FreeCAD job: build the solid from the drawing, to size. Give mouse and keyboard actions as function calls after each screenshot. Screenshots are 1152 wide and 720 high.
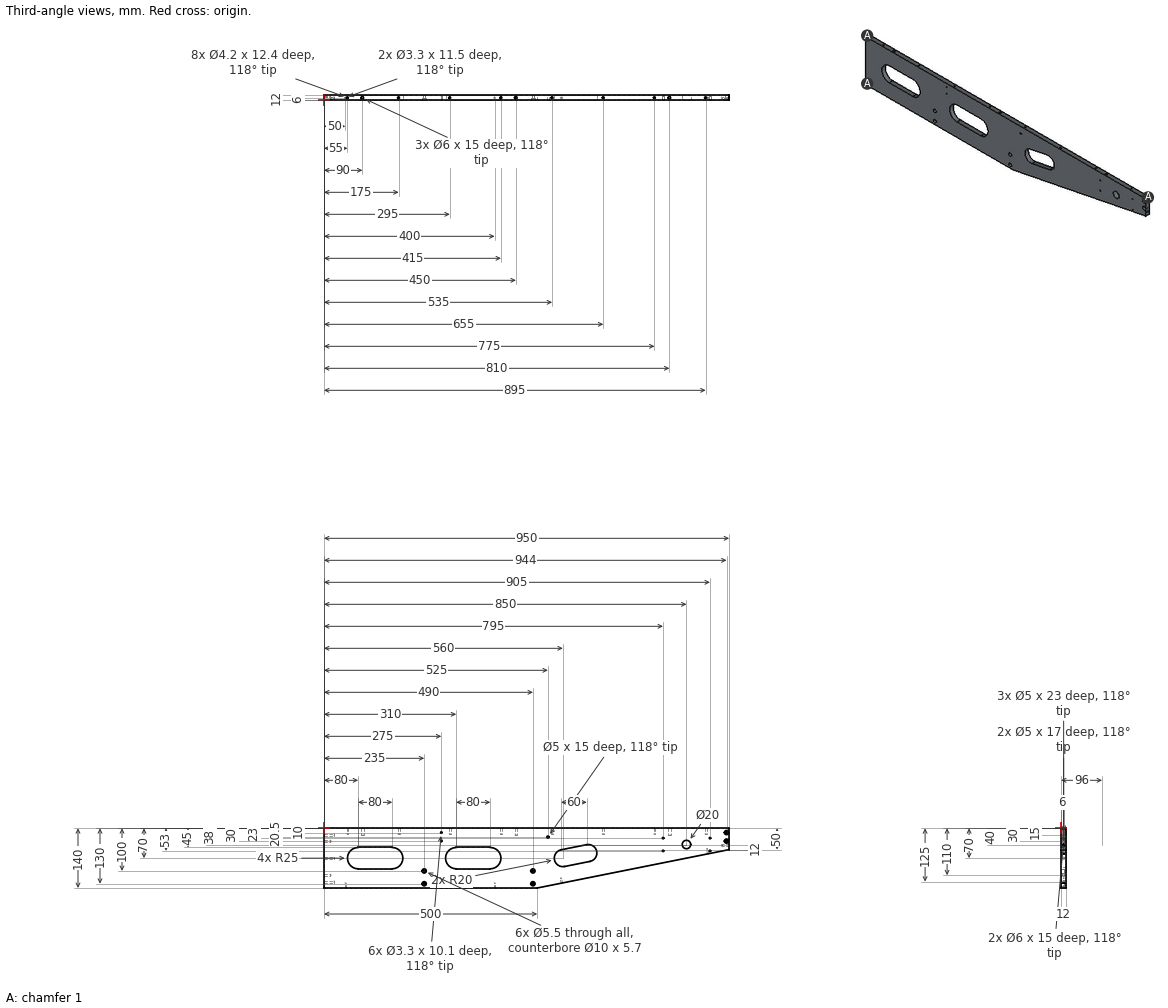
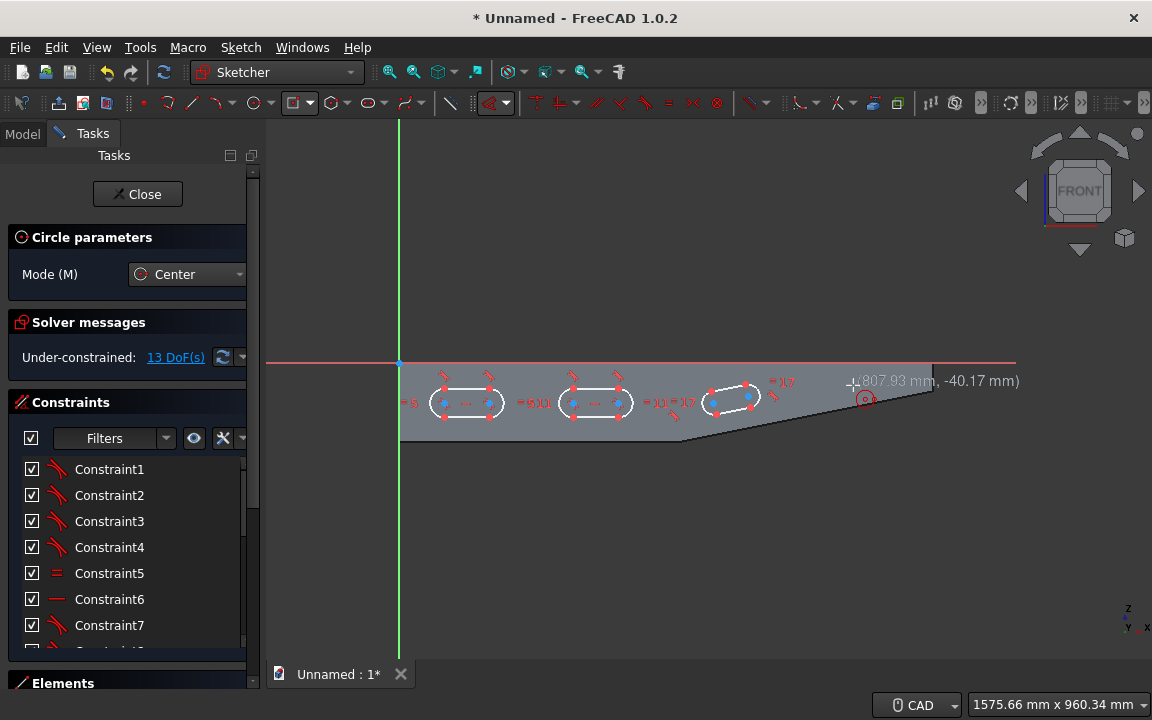
click(877, 384)
move(881, 380)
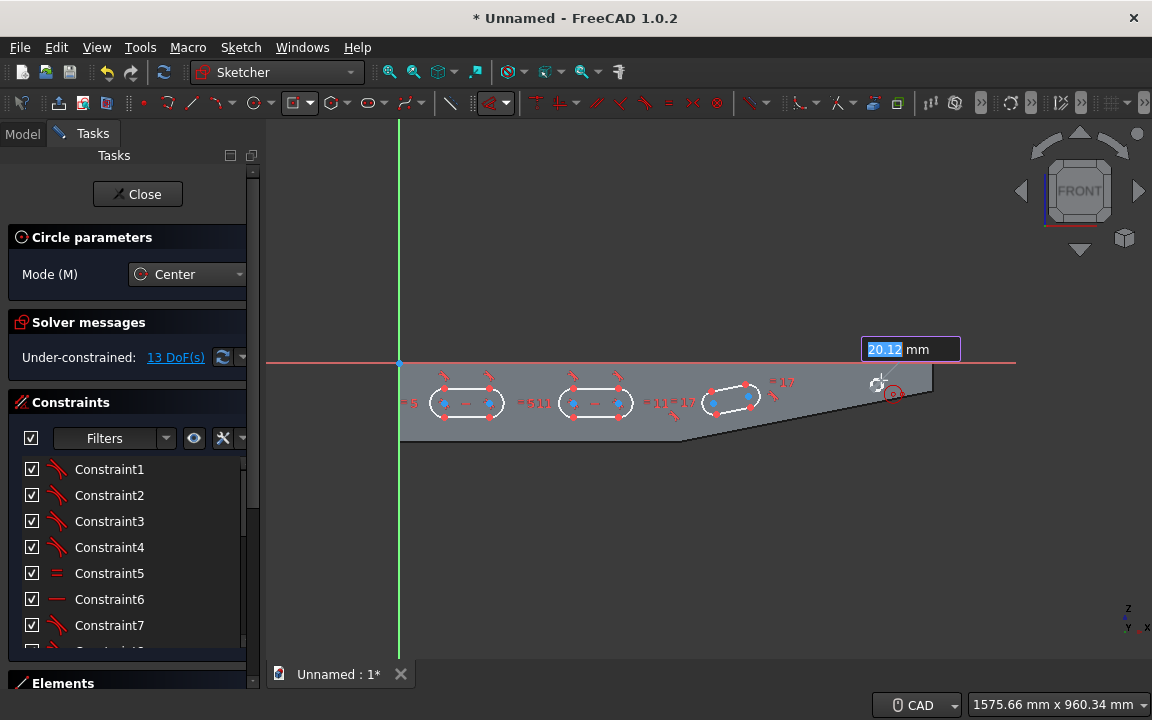
text(20)
key(Return)
key(Escape)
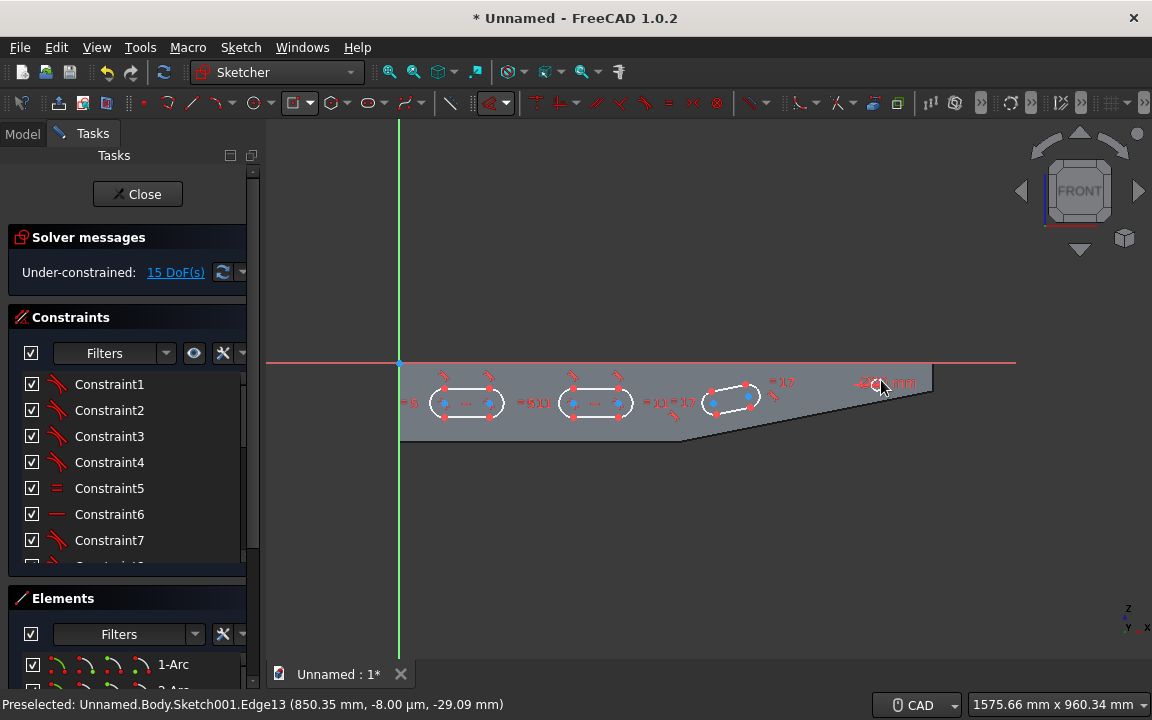
click(433, 395)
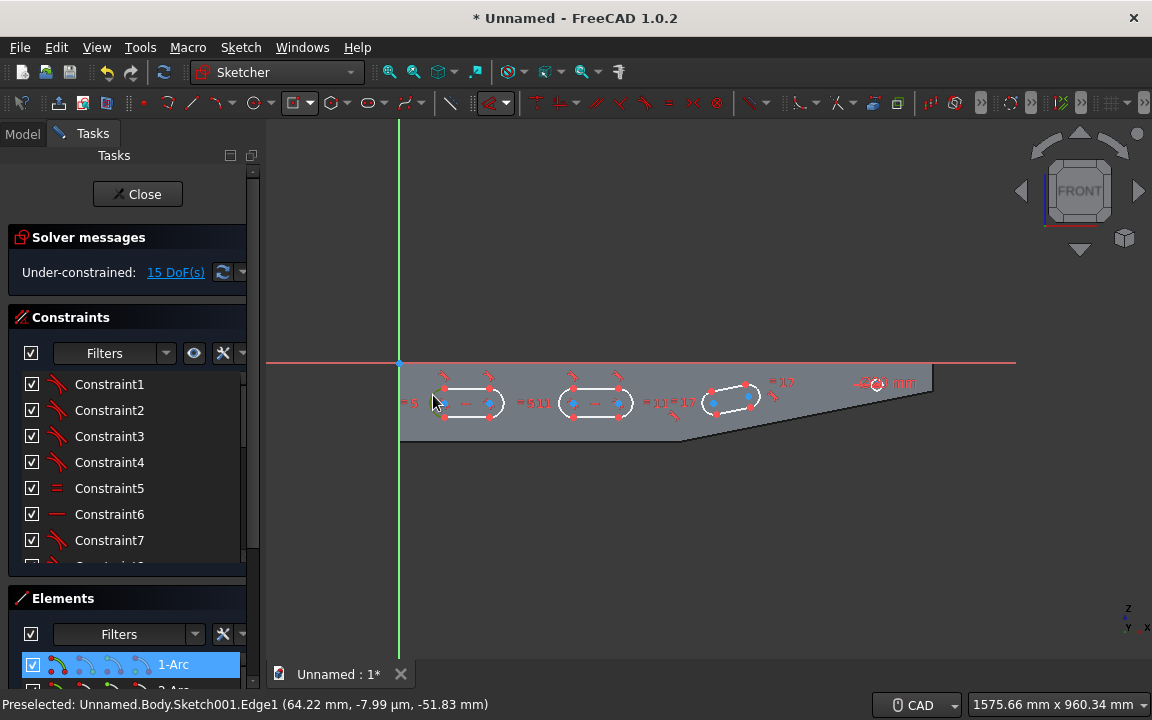
click(562, 395)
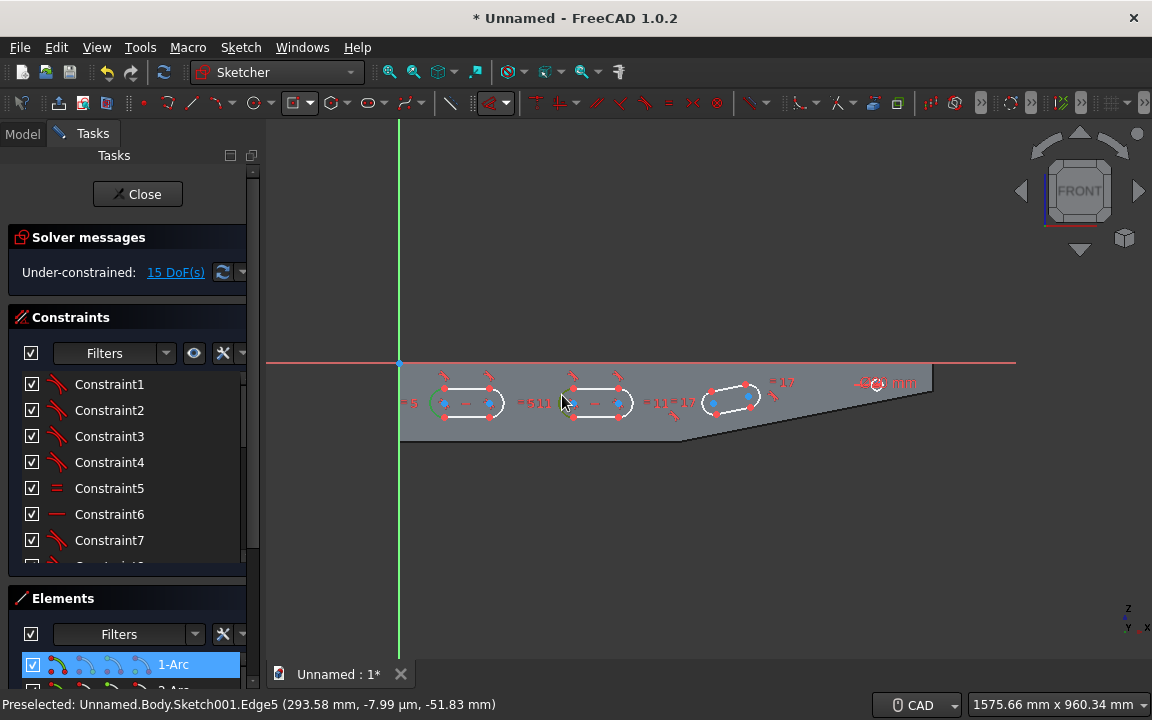
key(e)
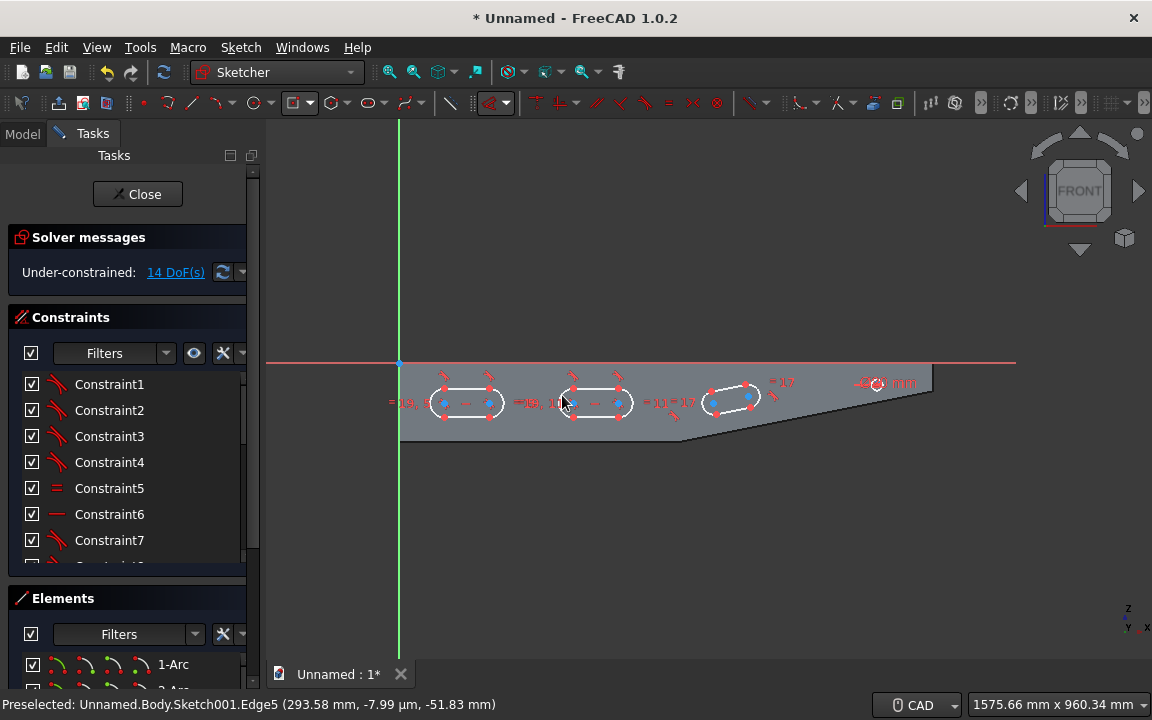
scroll(433, 395, up, 6)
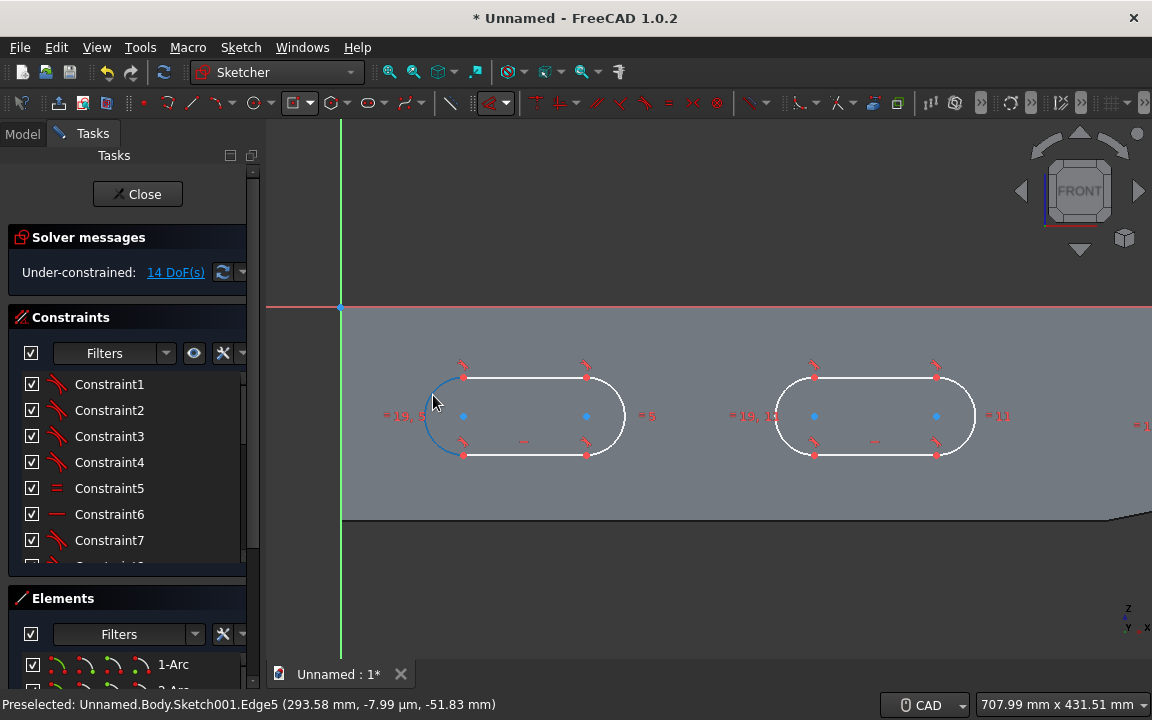
click(432, 393)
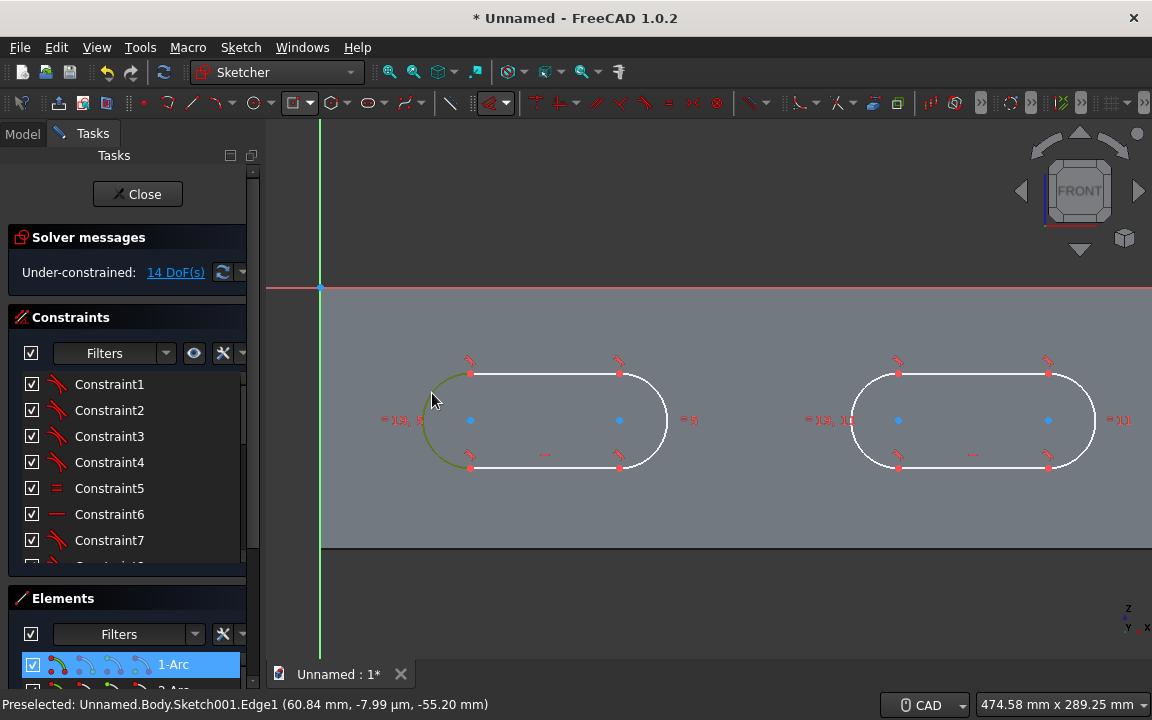
key(k)
key(r)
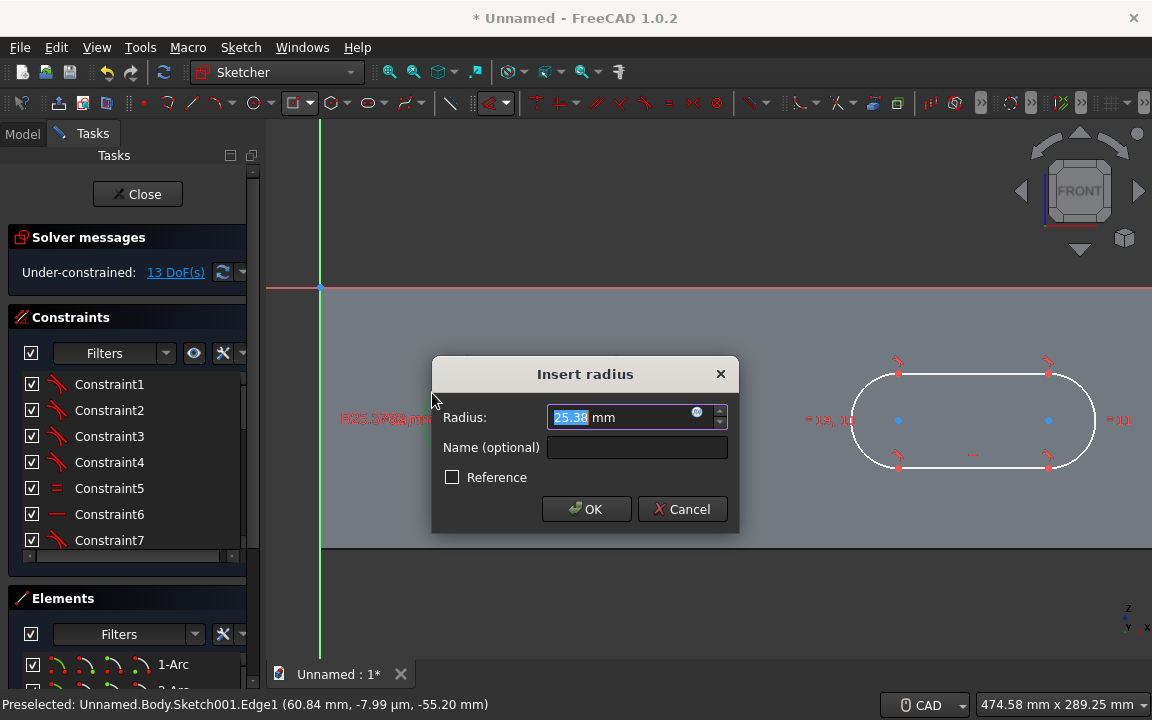
text(25)
key(Return)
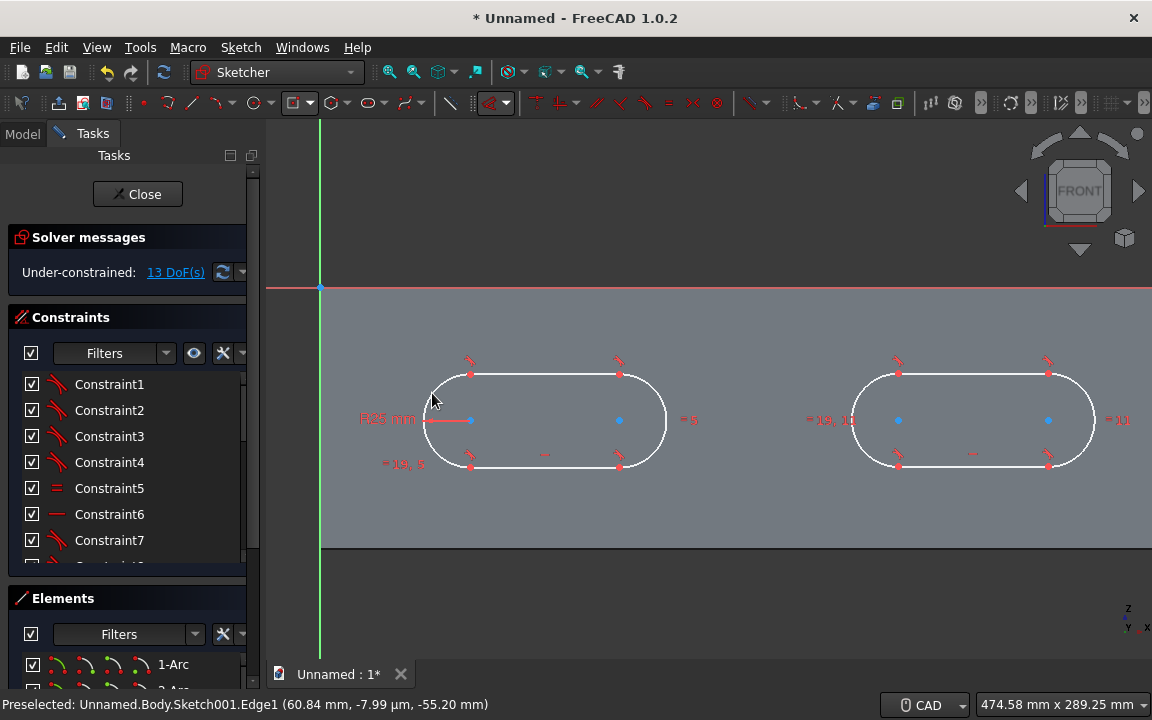
scroll(432, 394, down, 6)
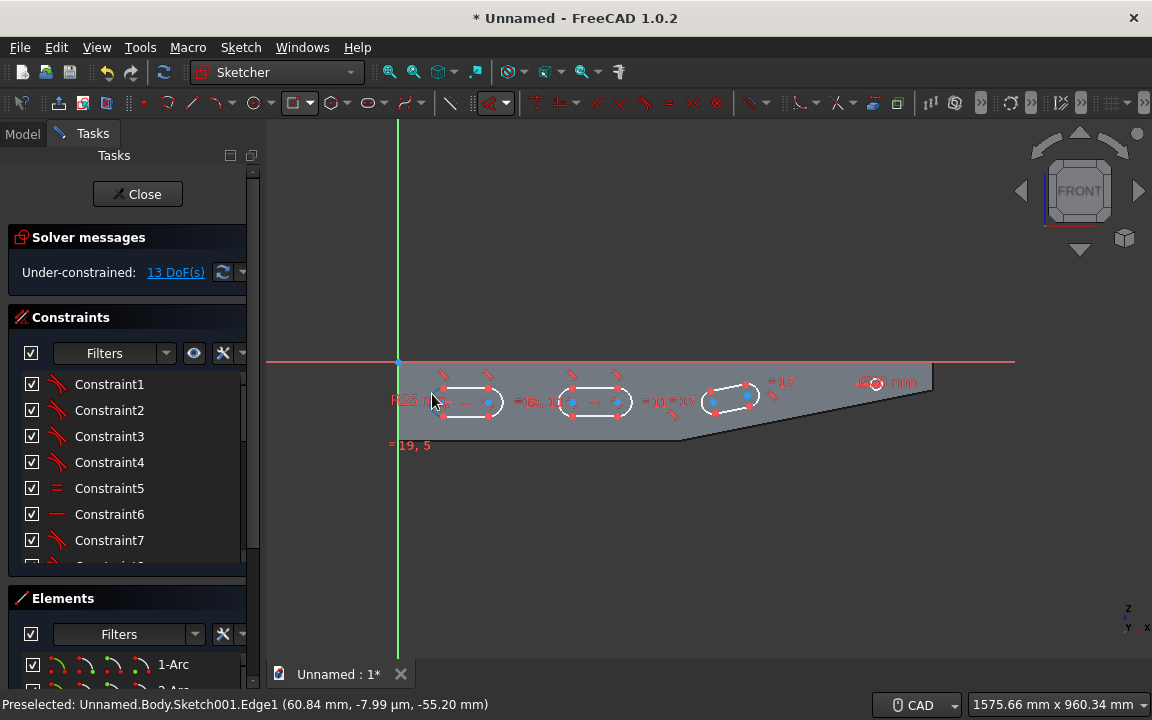
scroll(703, 398, up, 7)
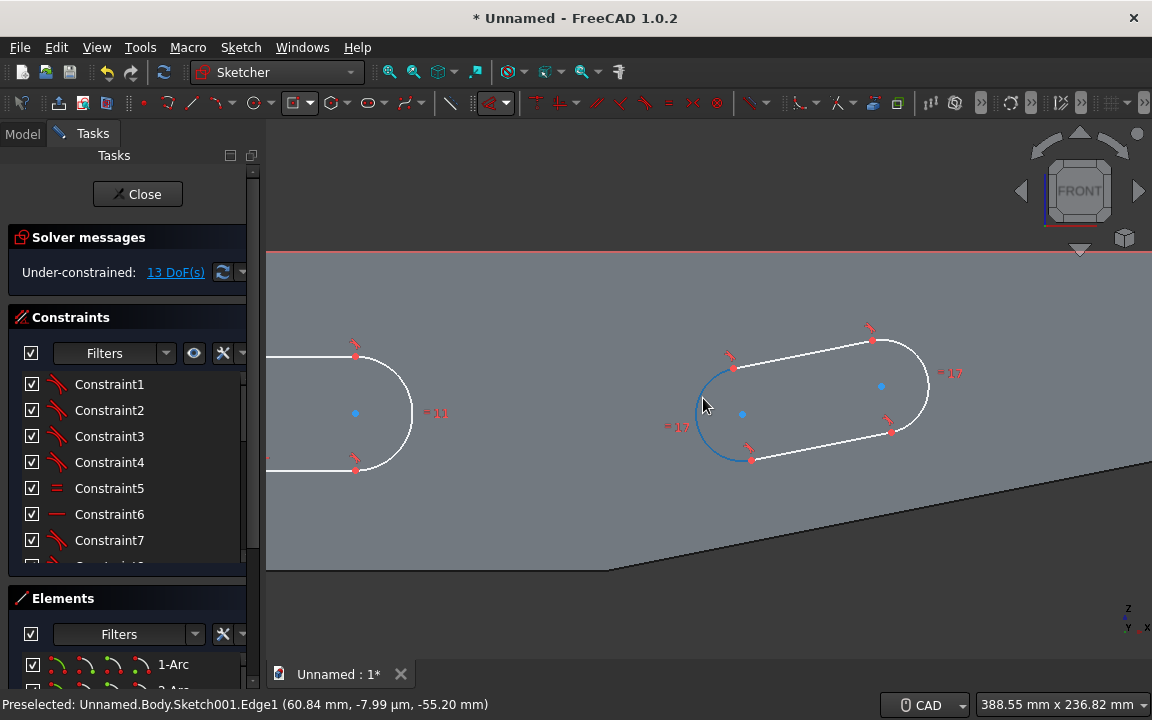
click(700, 395)